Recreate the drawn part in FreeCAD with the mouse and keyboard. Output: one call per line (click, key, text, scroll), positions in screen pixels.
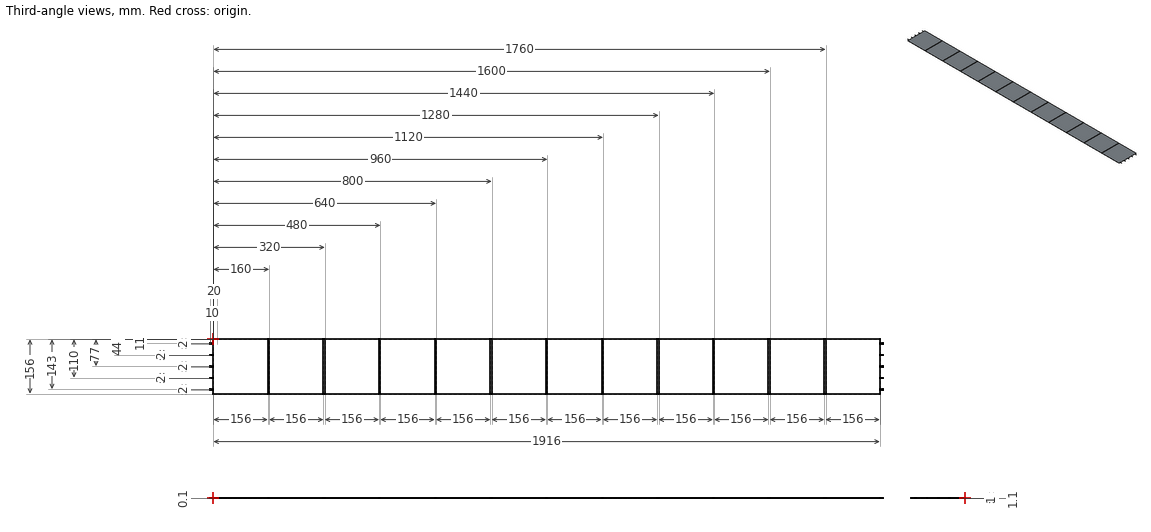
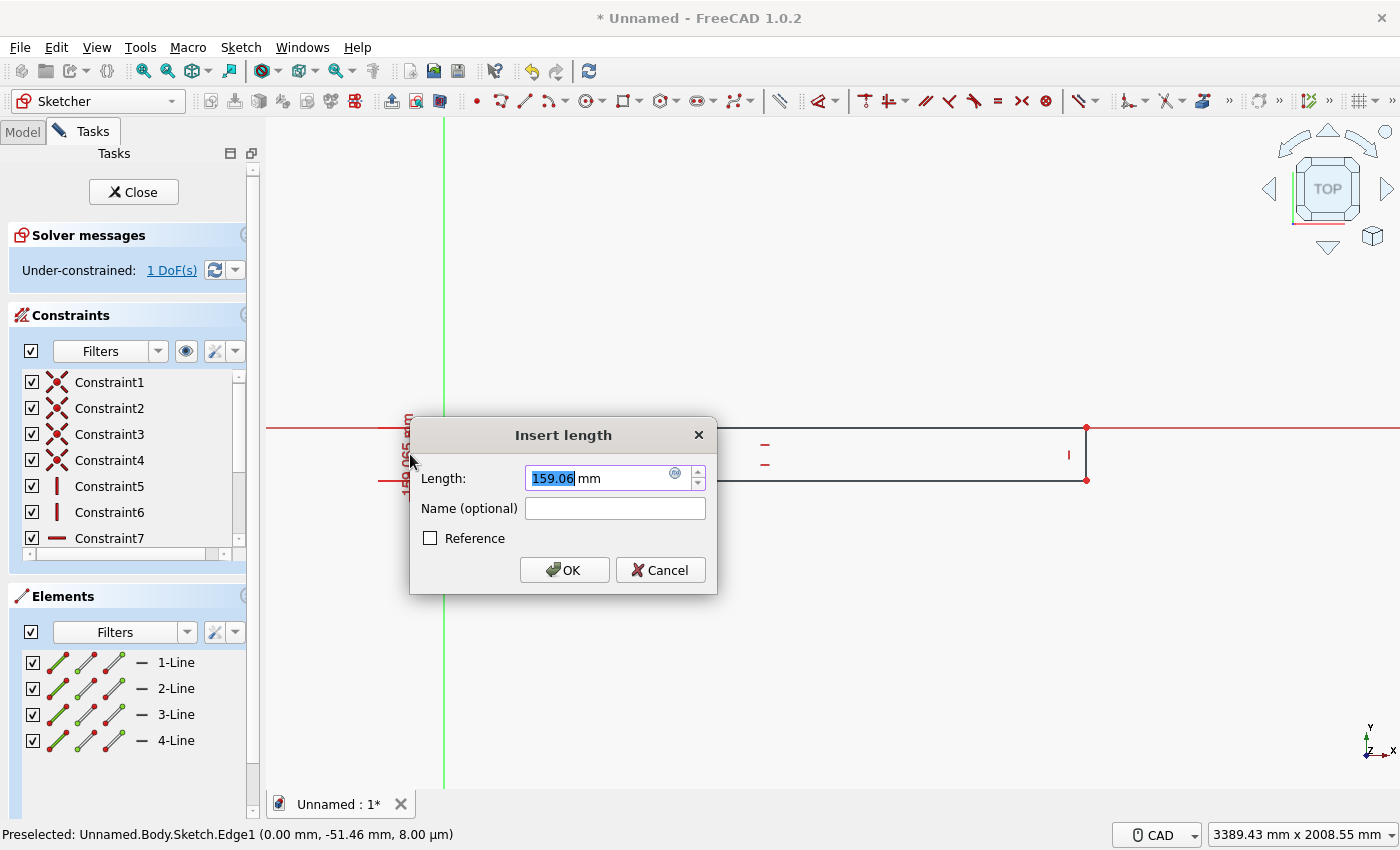
text(156)
key(Return)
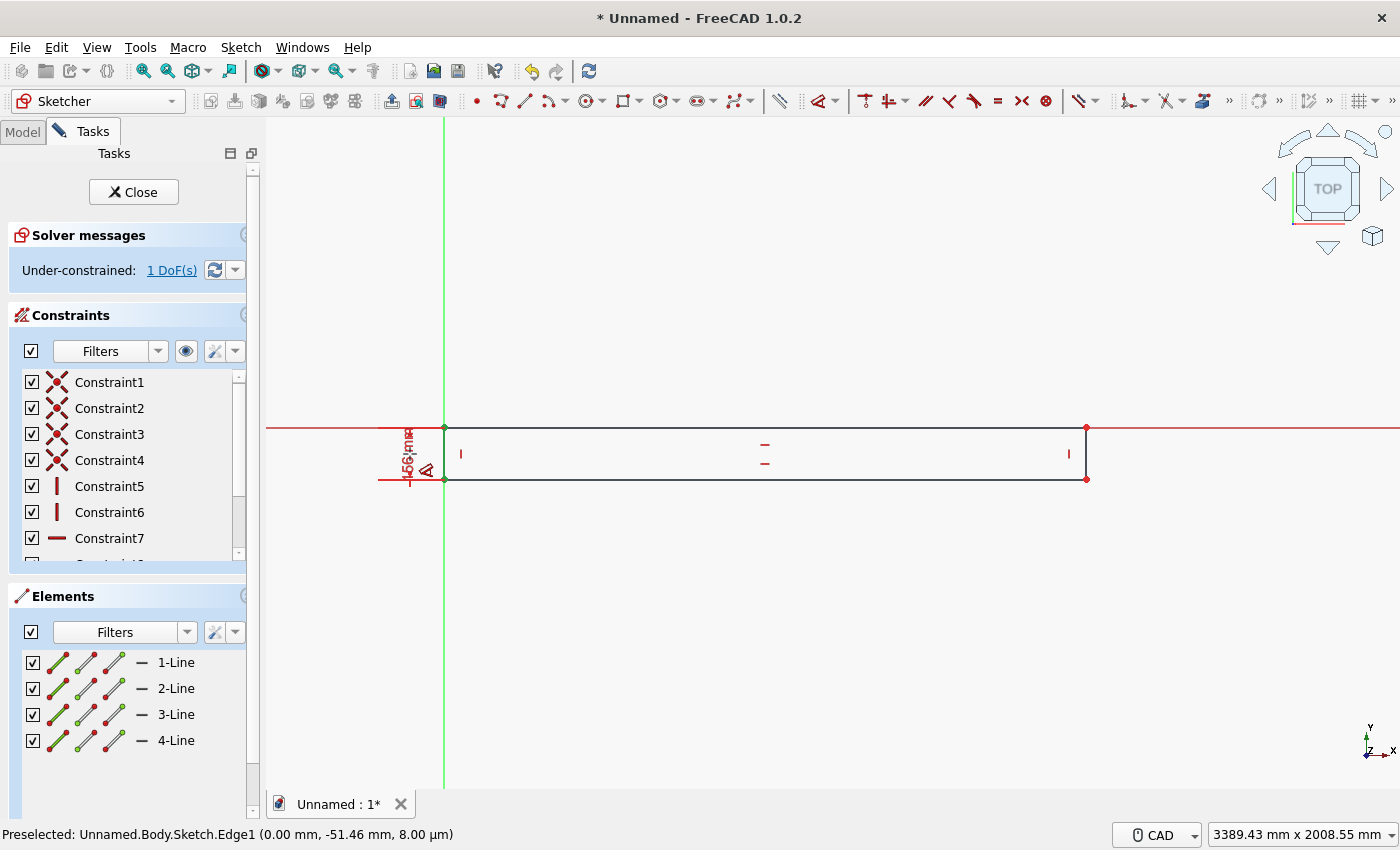
click(637, 480)
click(765, 514)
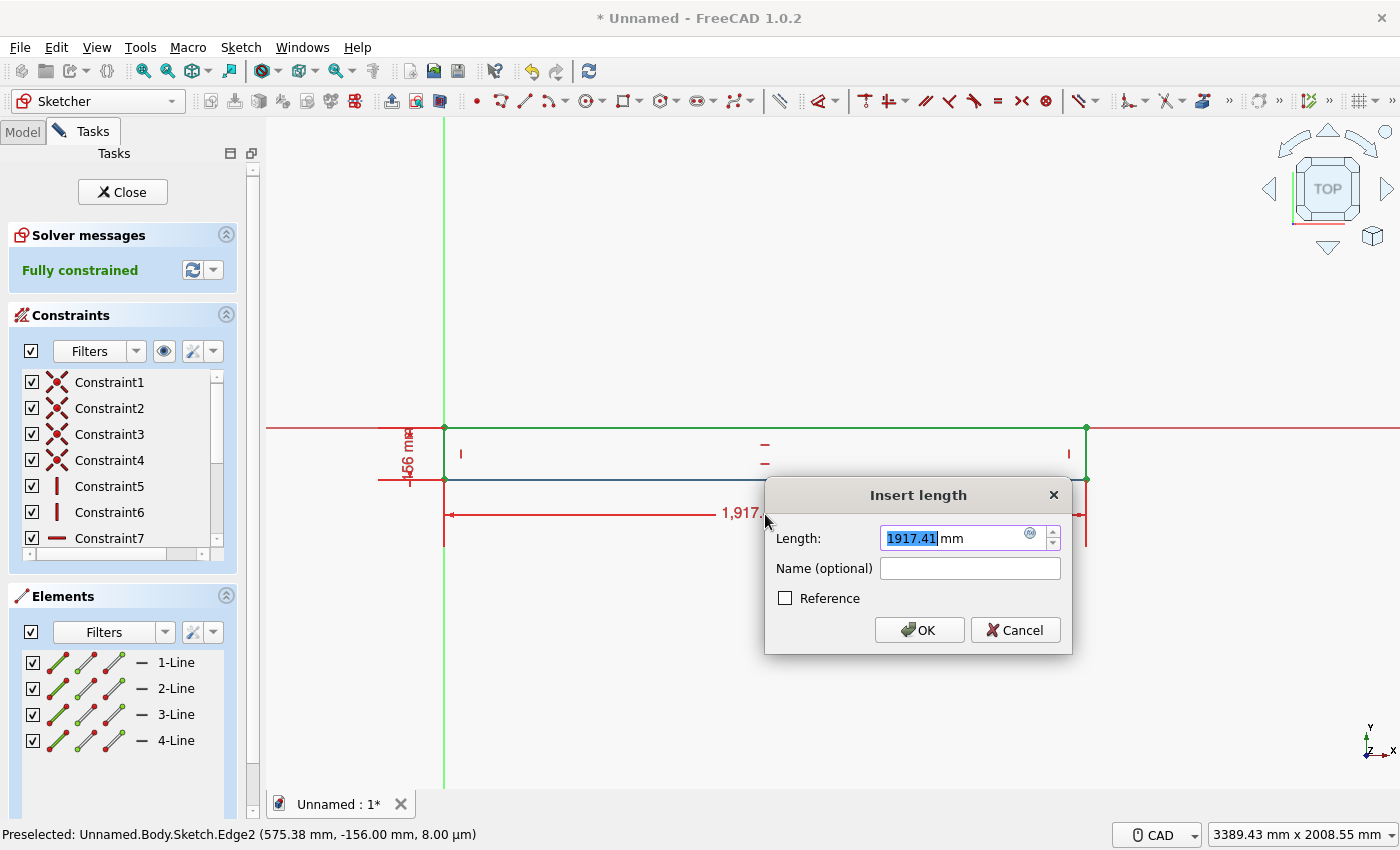
text(1916)
key(Return)
key(Escape)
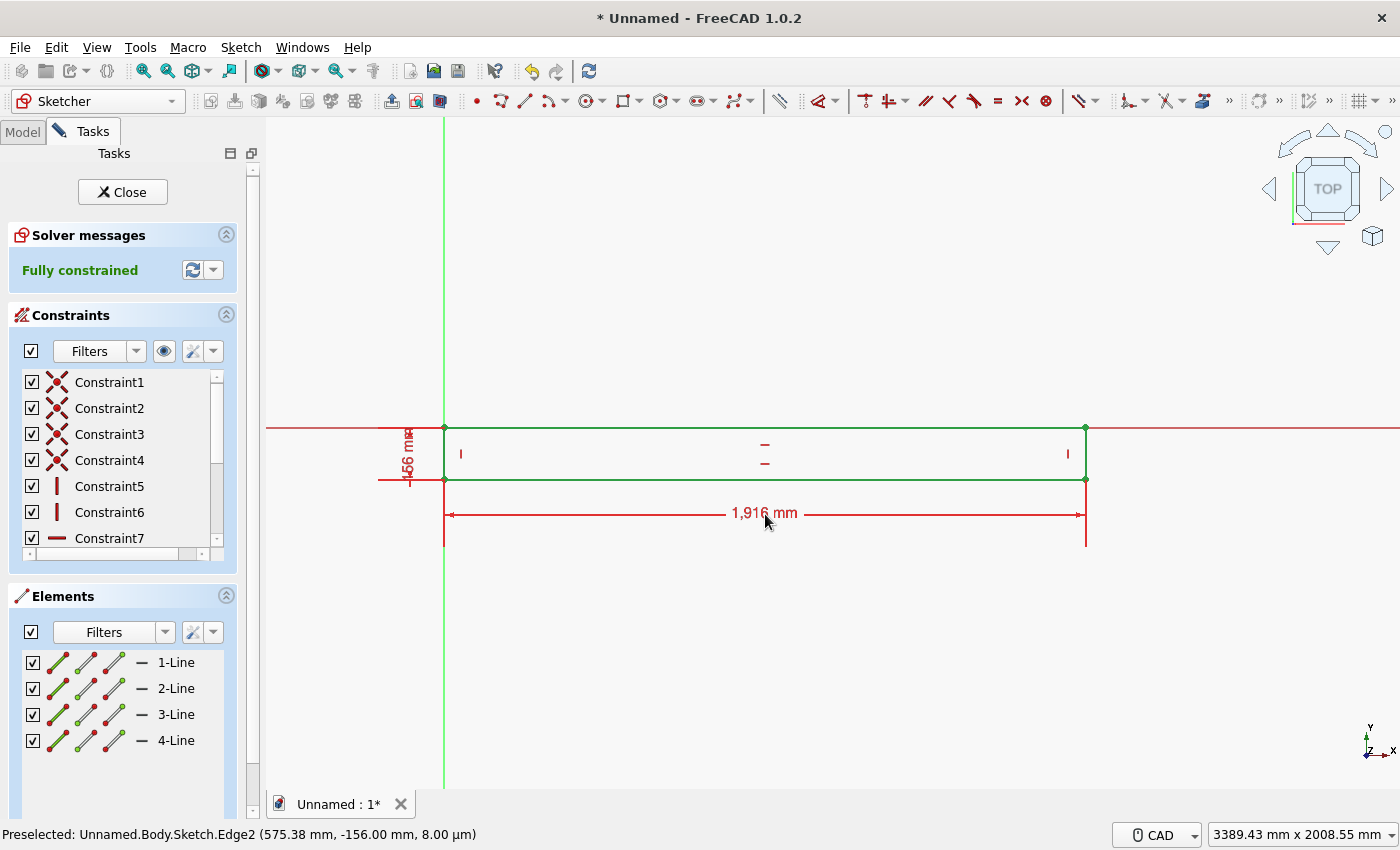
click(123, 192)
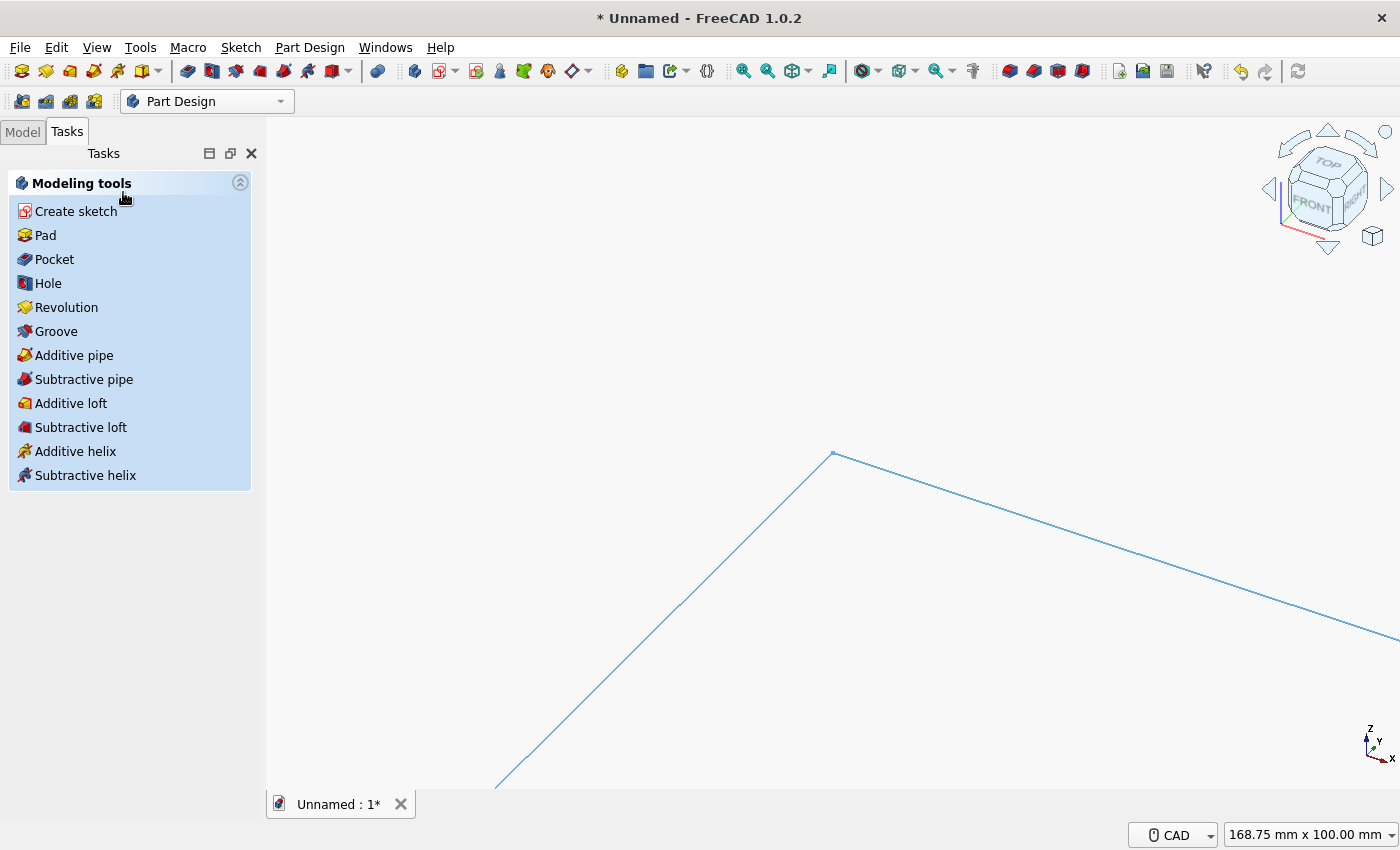
click(22, 72)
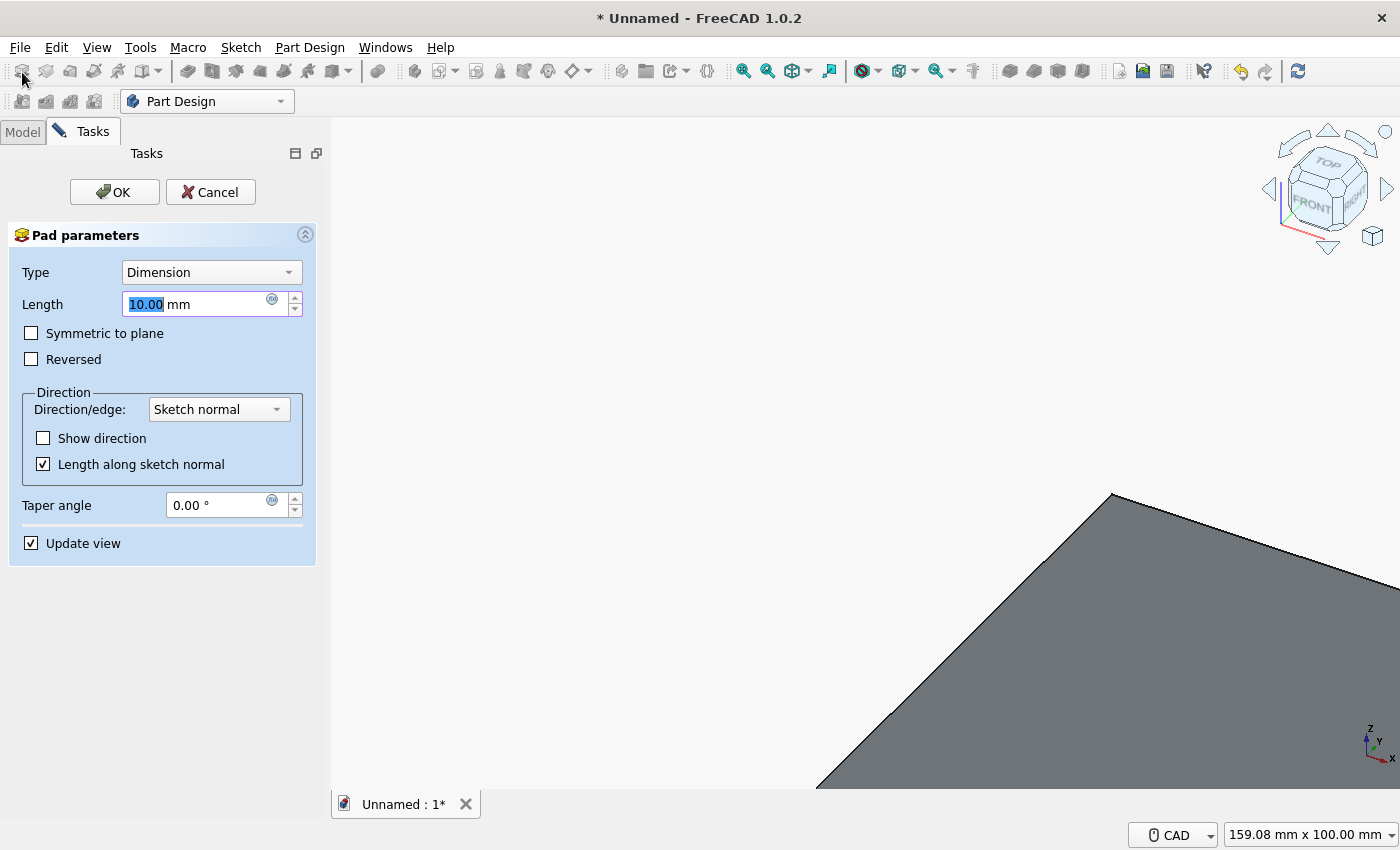
text(1)
key(Tab)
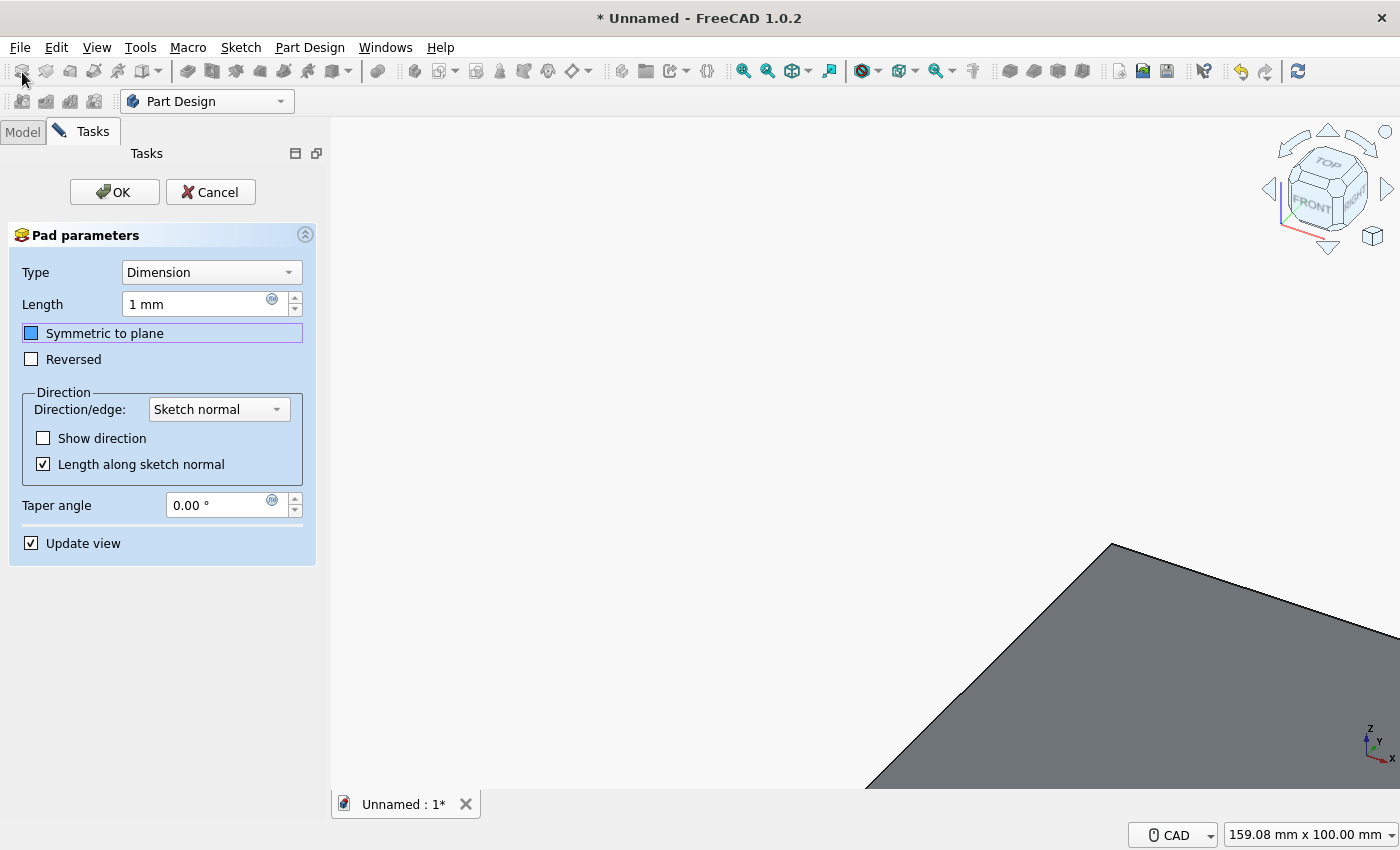
click(115, 192)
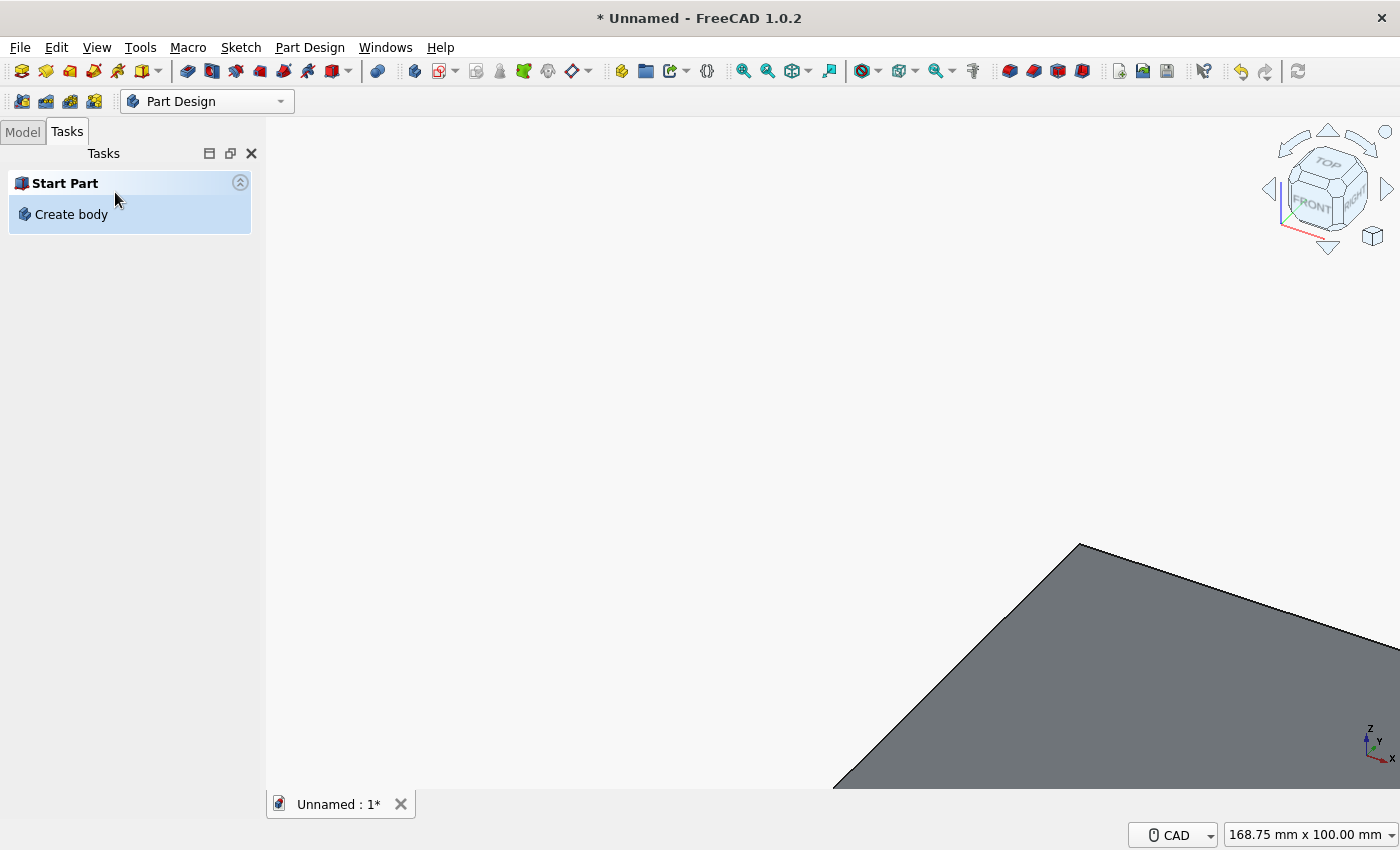
key(v)
key(f)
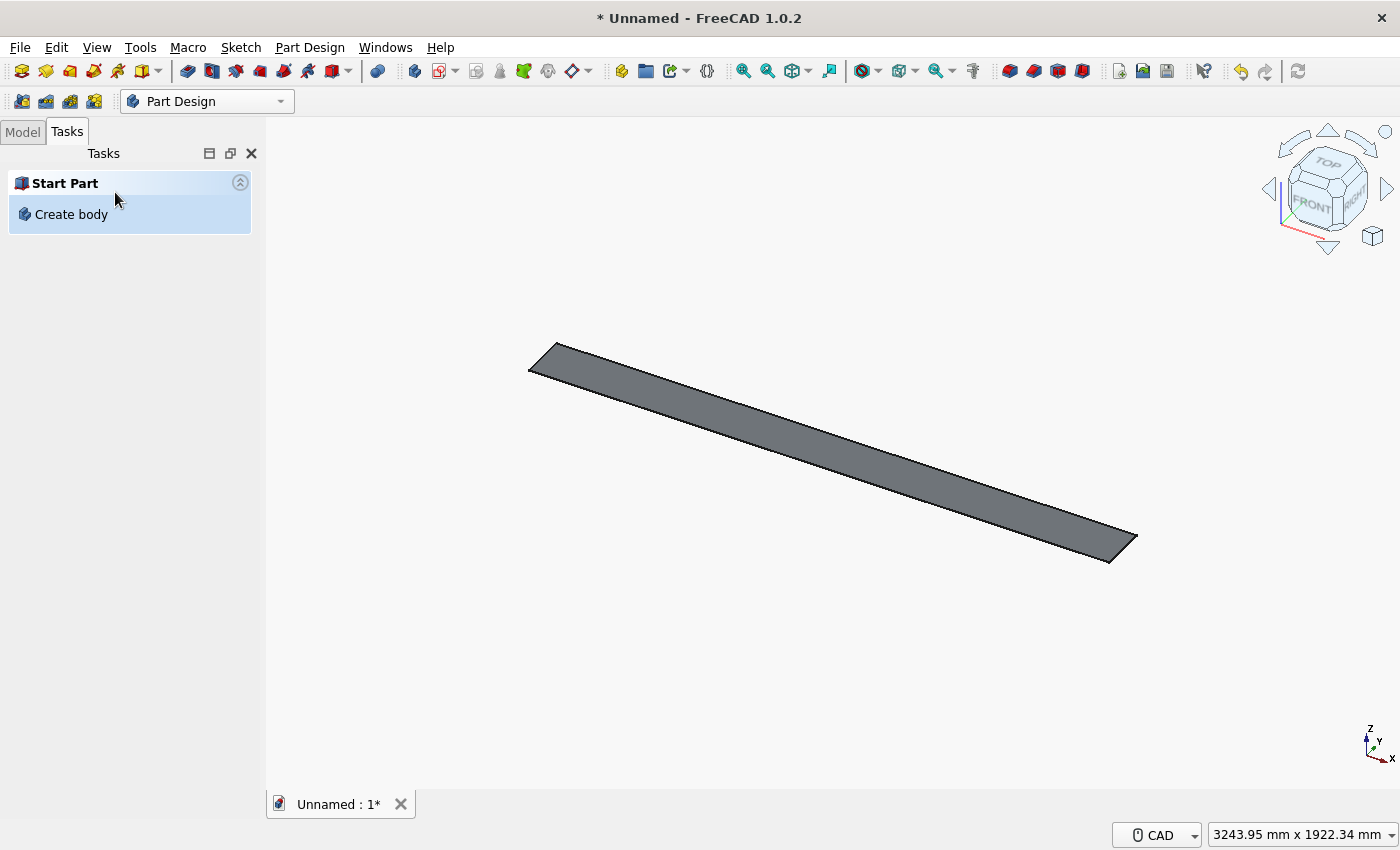
click(1082, 534)